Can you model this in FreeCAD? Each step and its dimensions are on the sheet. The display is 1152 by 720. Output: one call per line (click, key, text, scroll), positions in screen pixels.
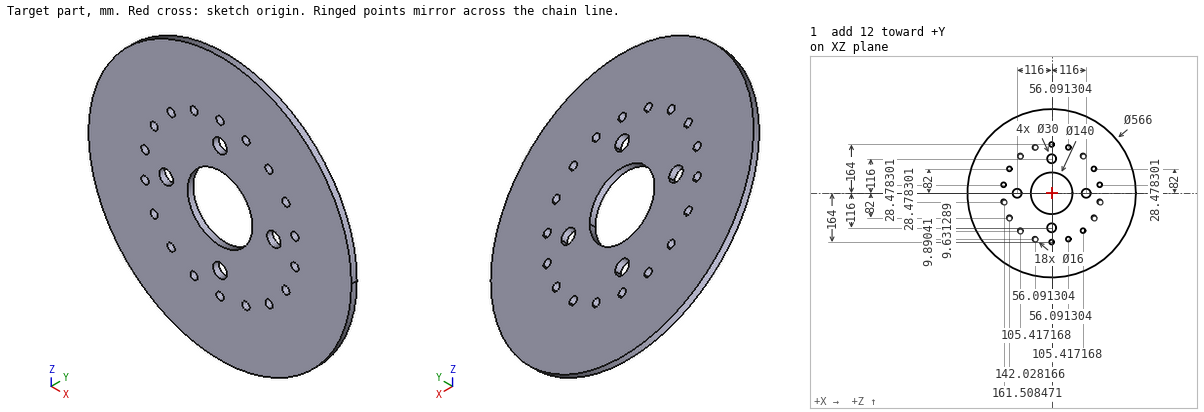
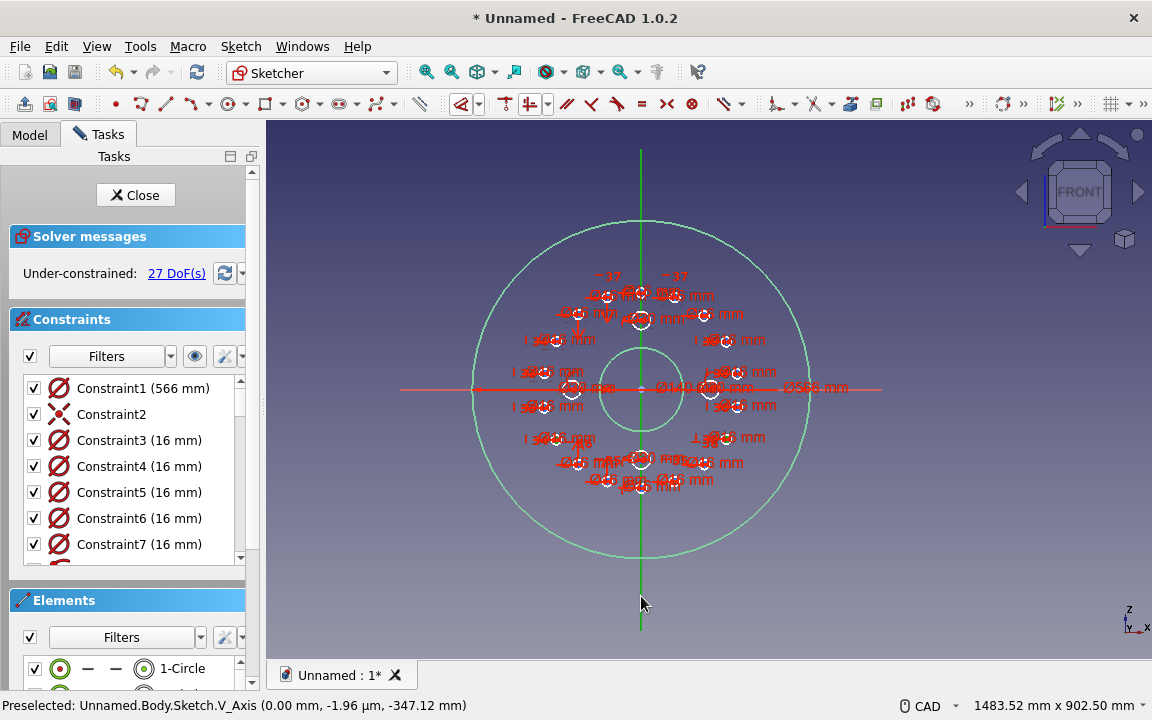
click(667, 104)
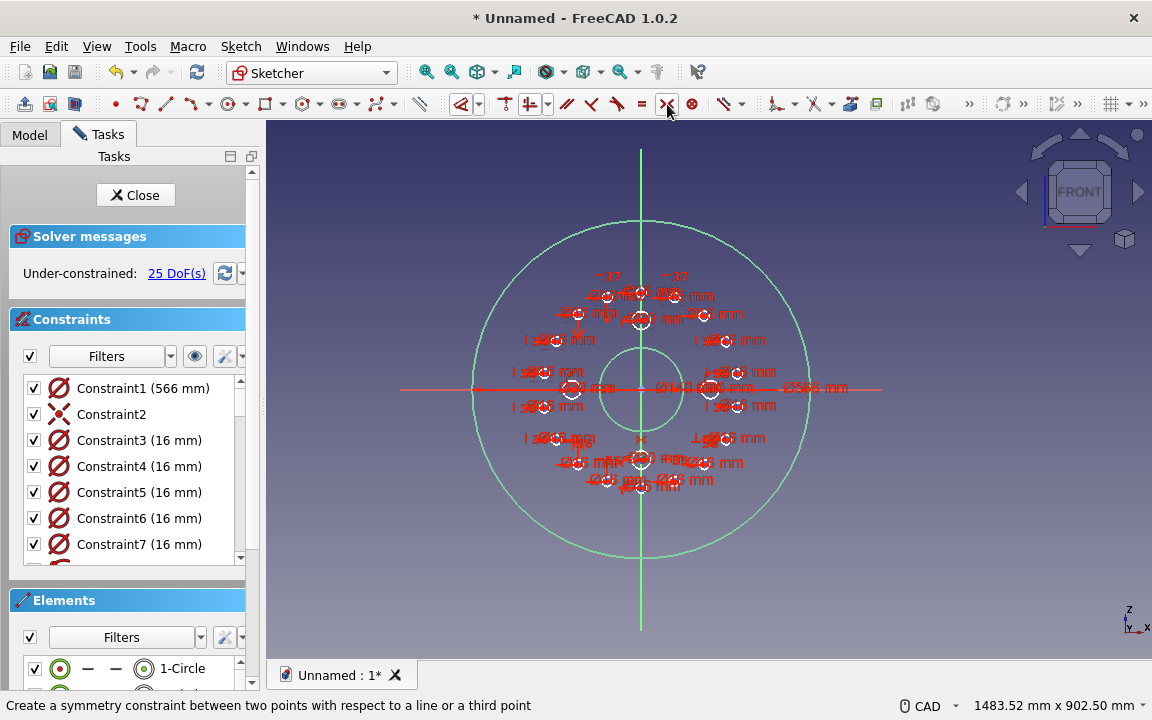
click(544, 408)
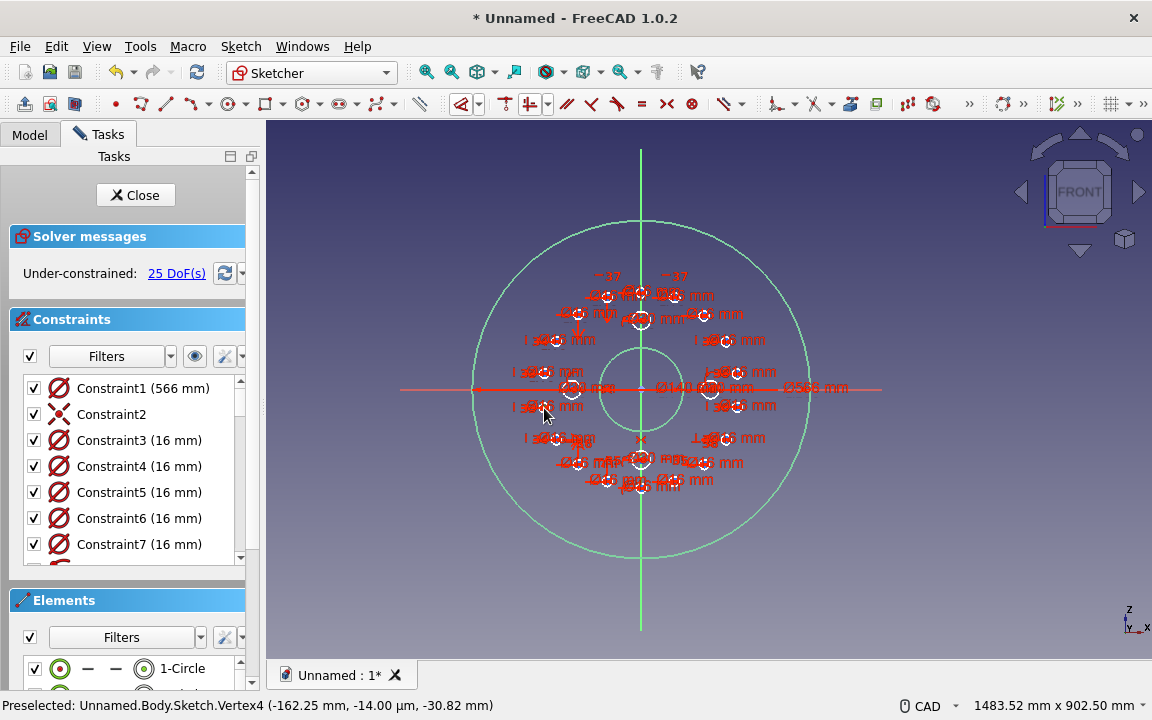
click(737, 407)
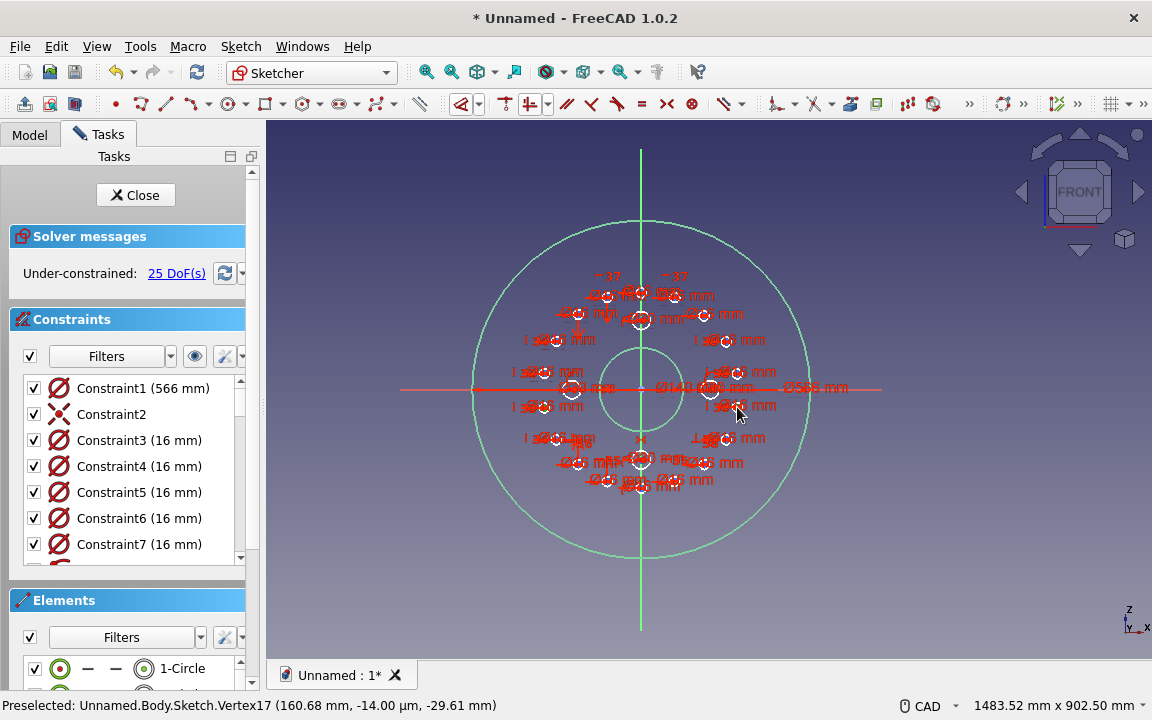
click(641, 596)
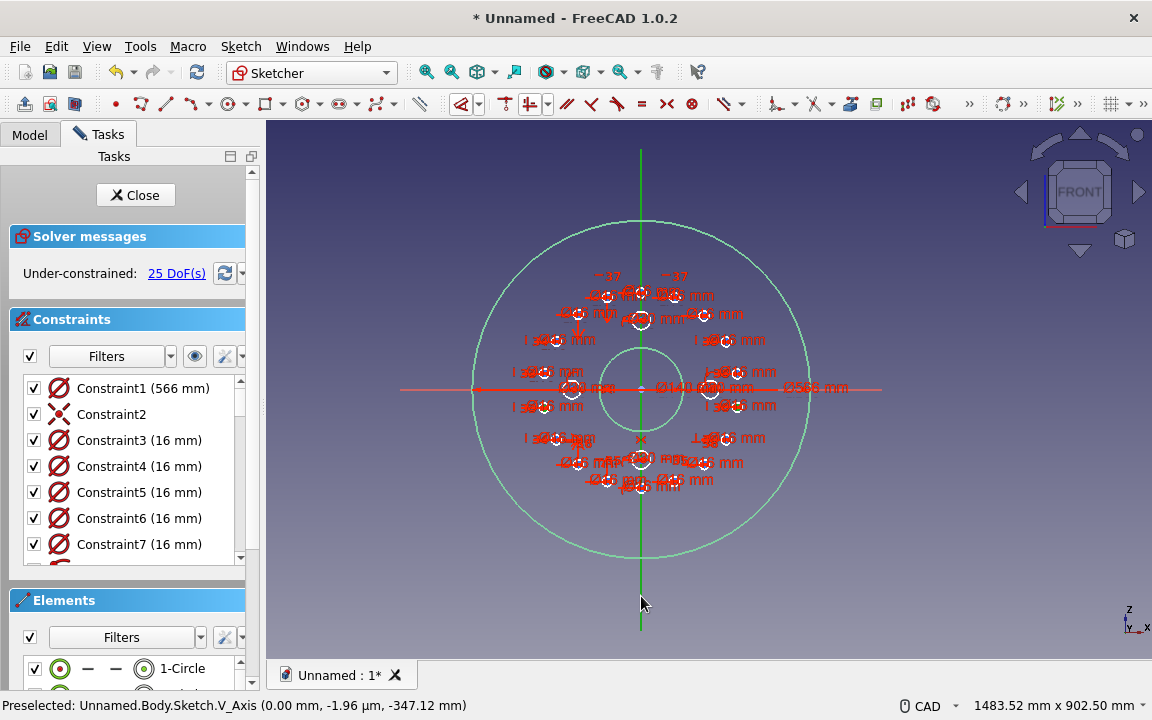
click(667, 104)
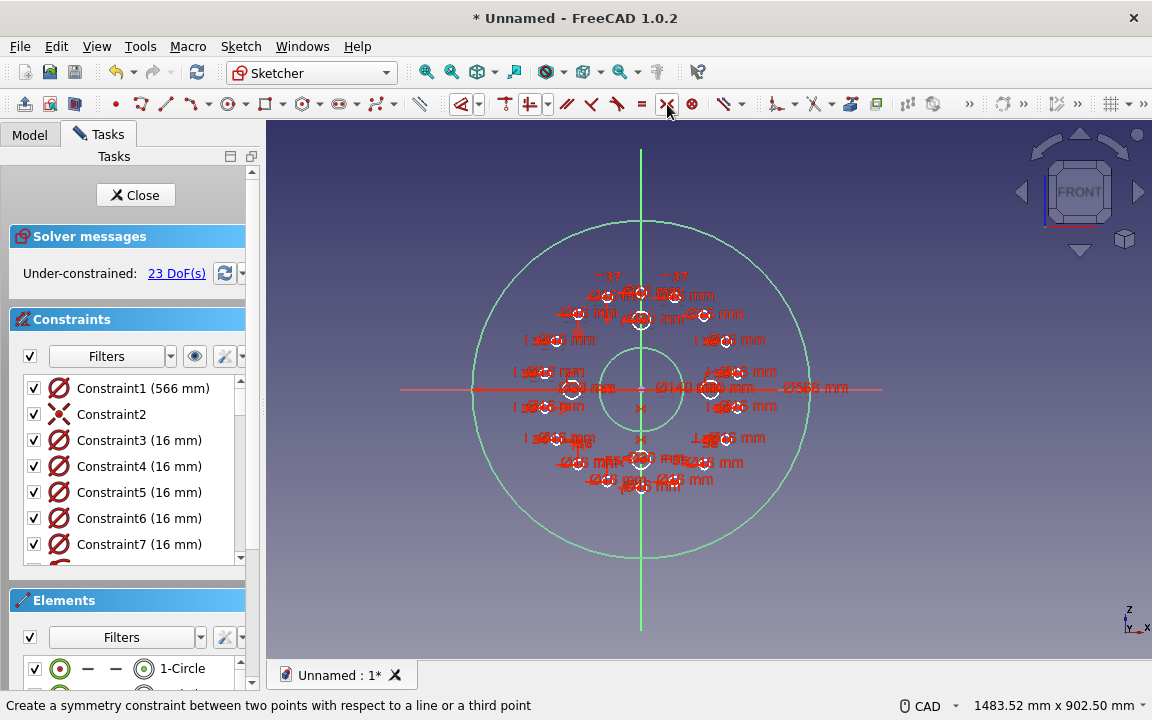
click(578, 315)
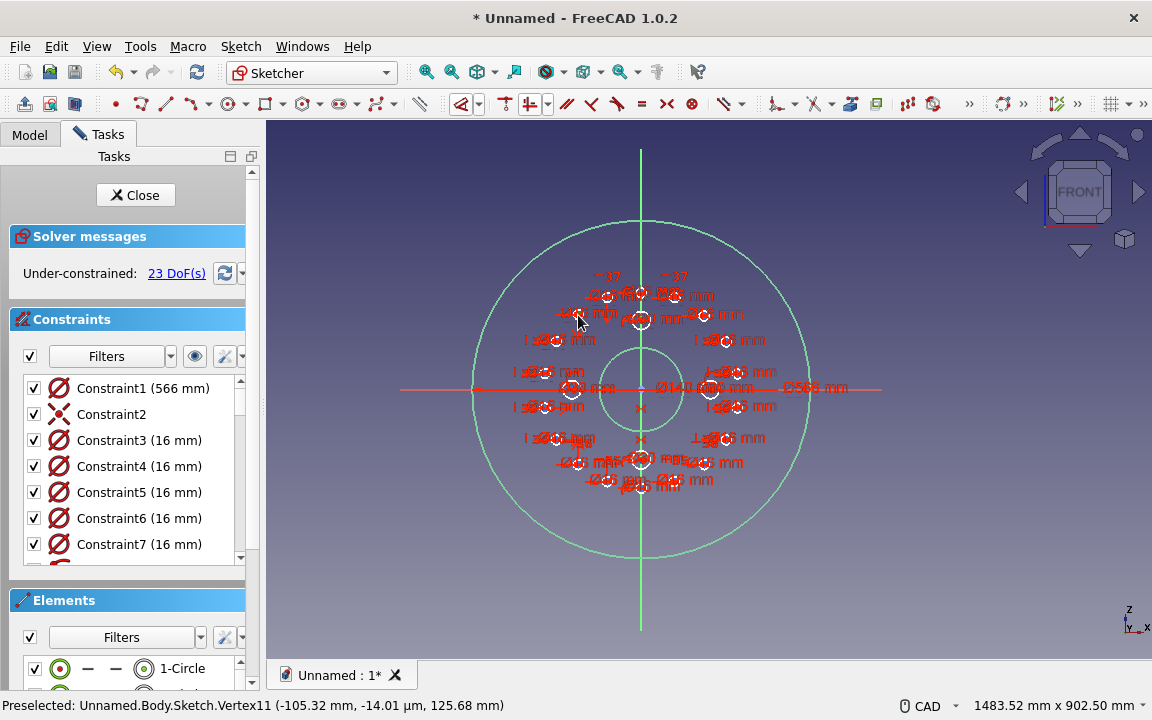
click(704, 316)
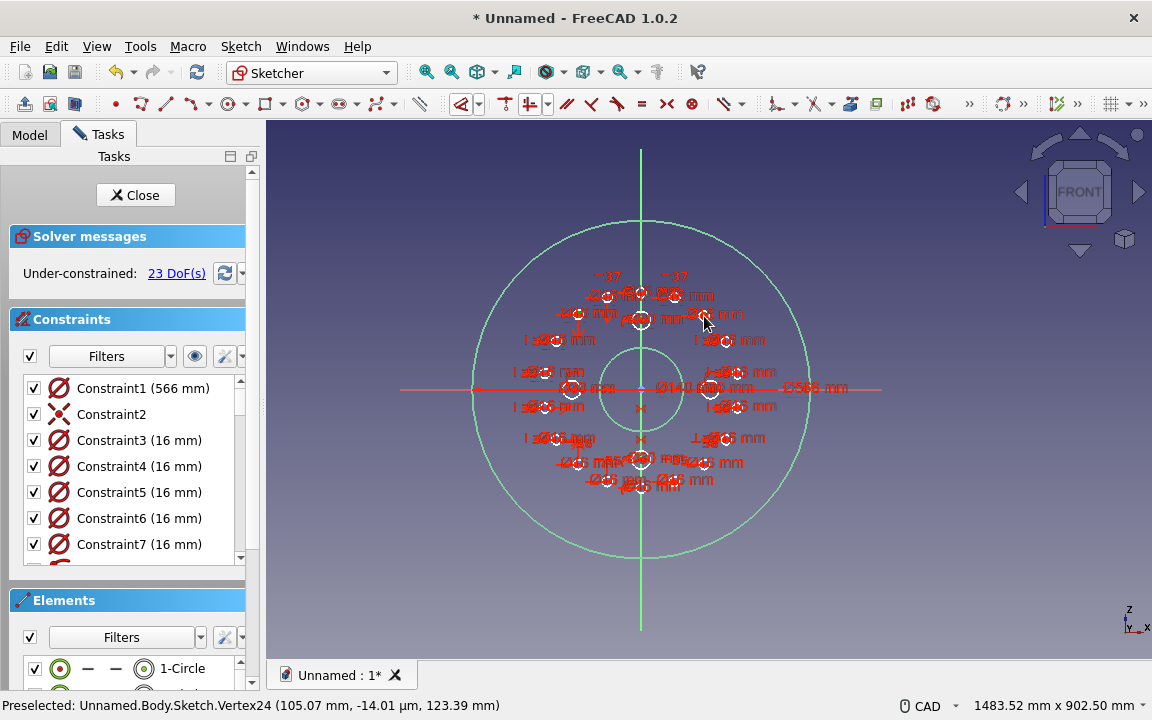
click(641, 596)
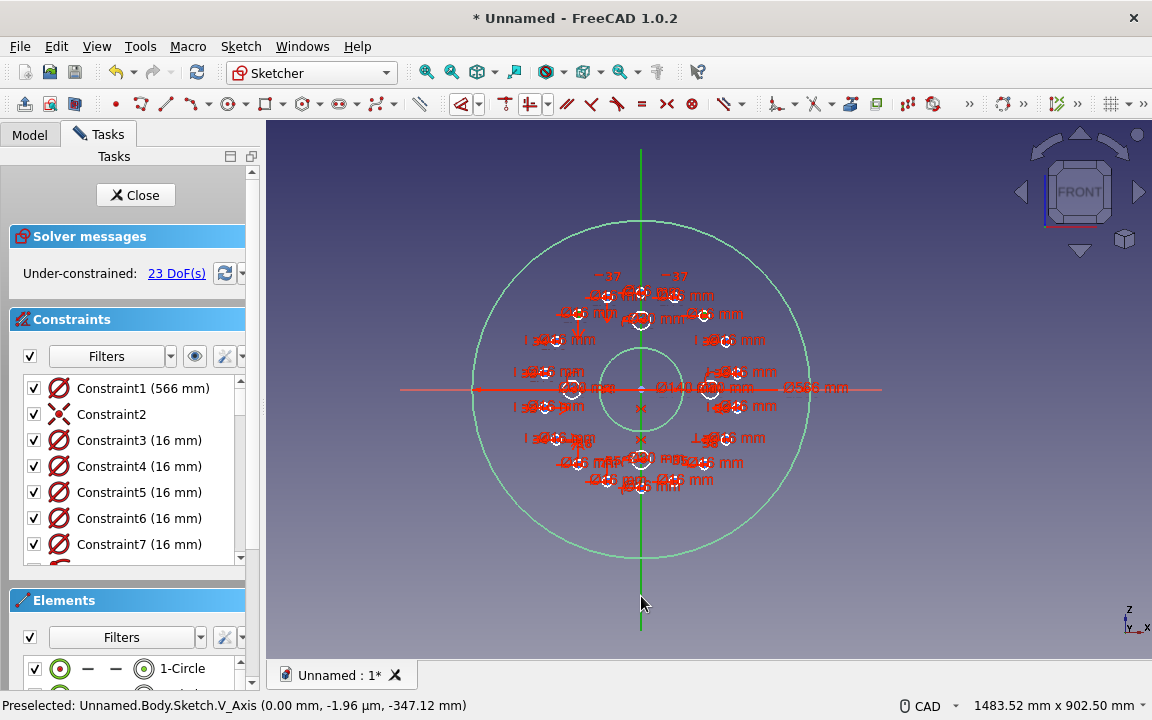
click(667, 104)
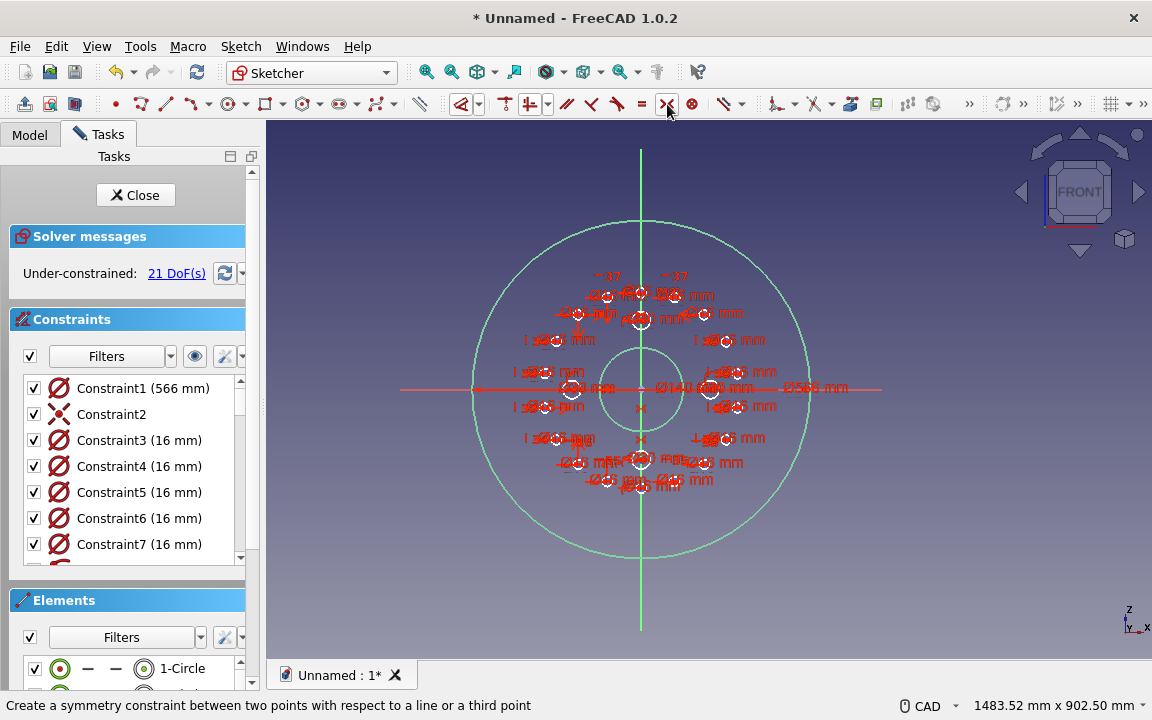
click(460, 104)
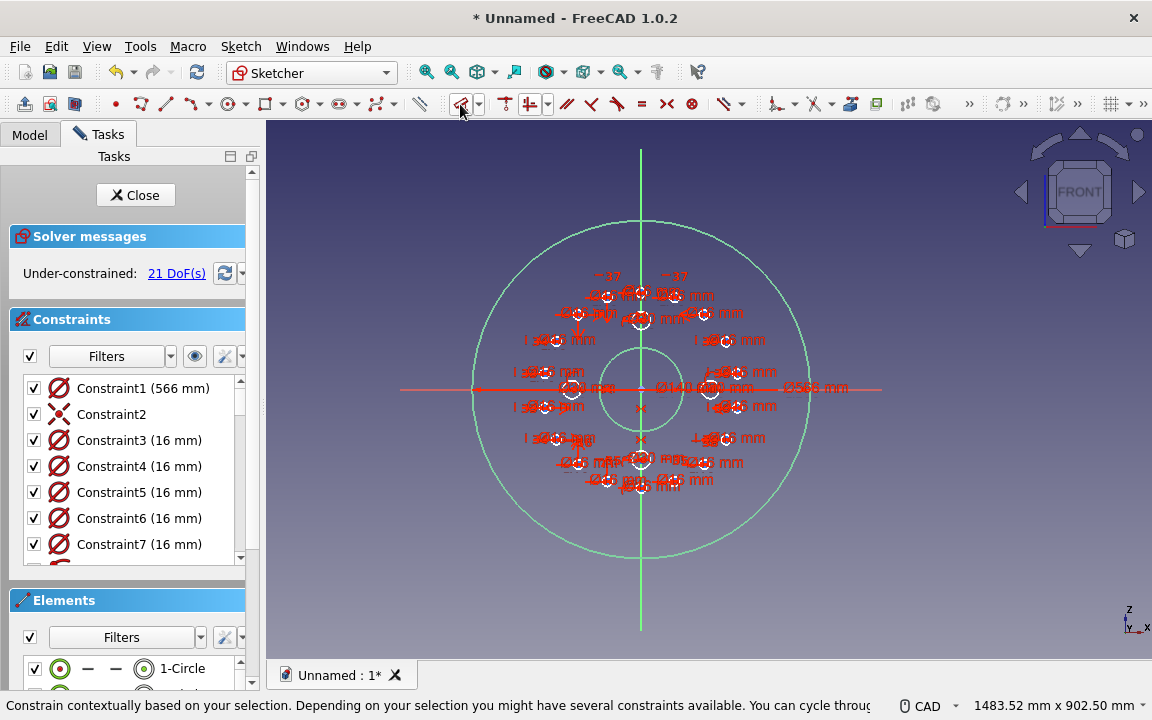
click(556, 440)
click(522, 415)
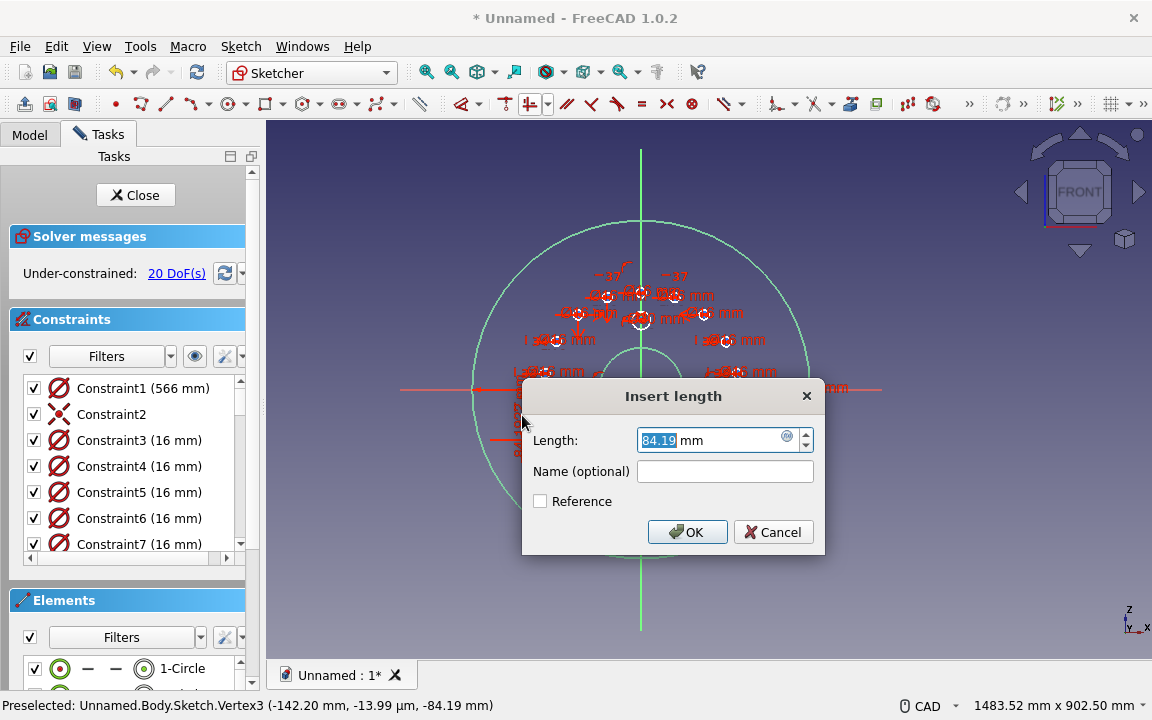
text(82)
key(Return)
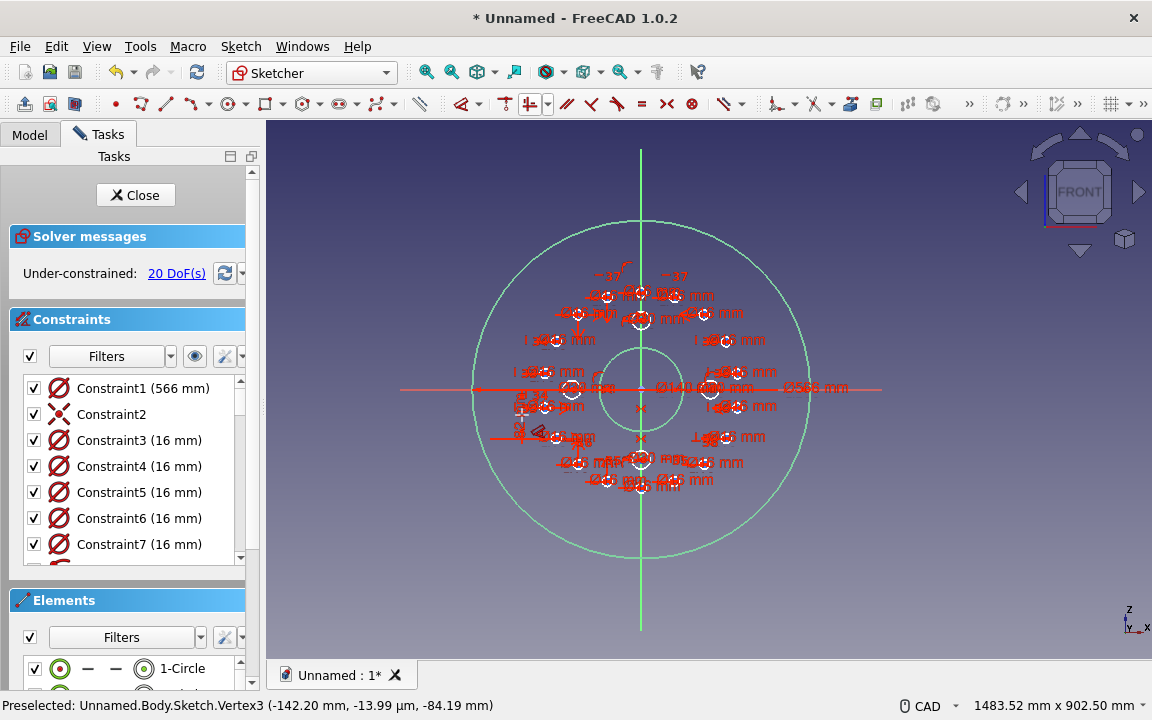
click(556, 342)
click(522, 366)